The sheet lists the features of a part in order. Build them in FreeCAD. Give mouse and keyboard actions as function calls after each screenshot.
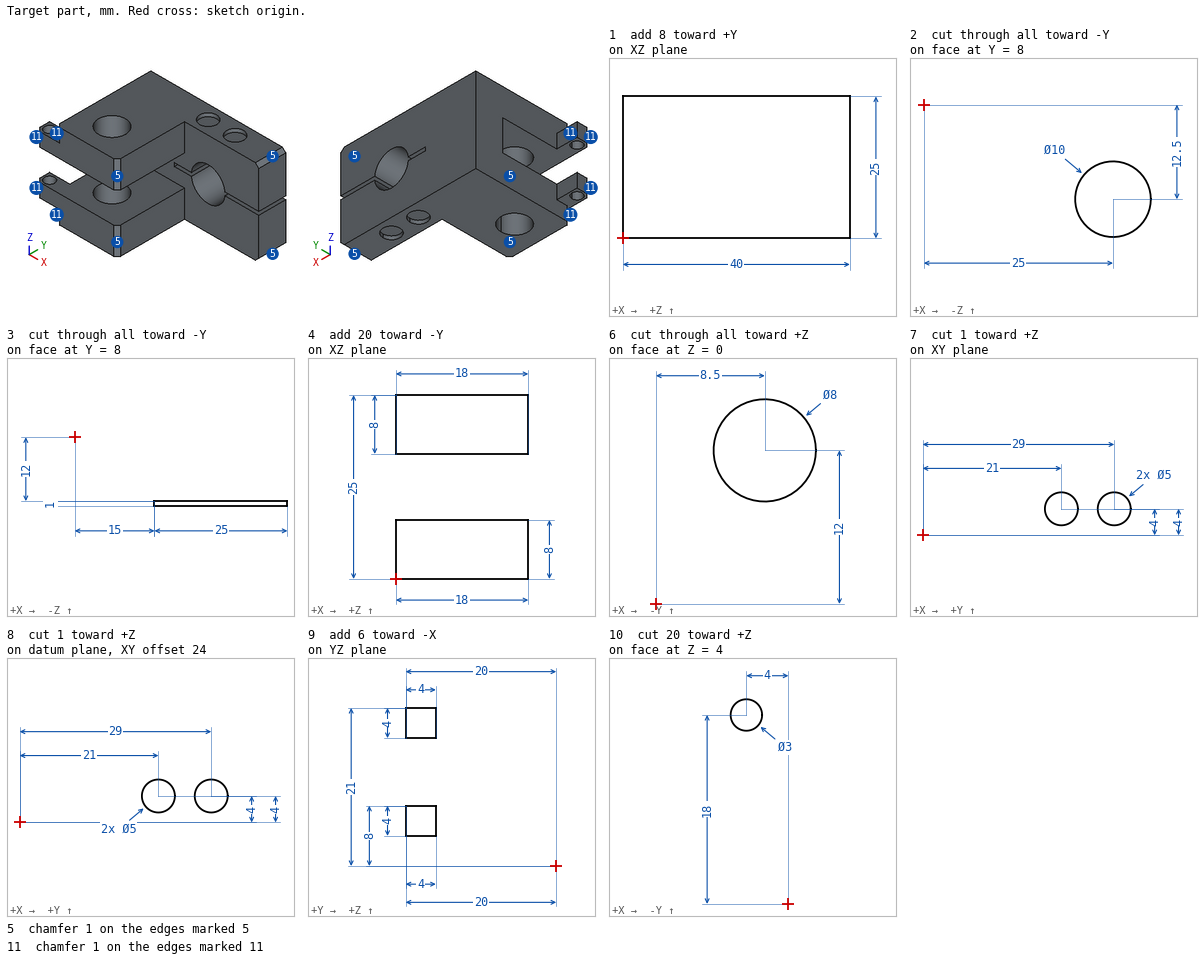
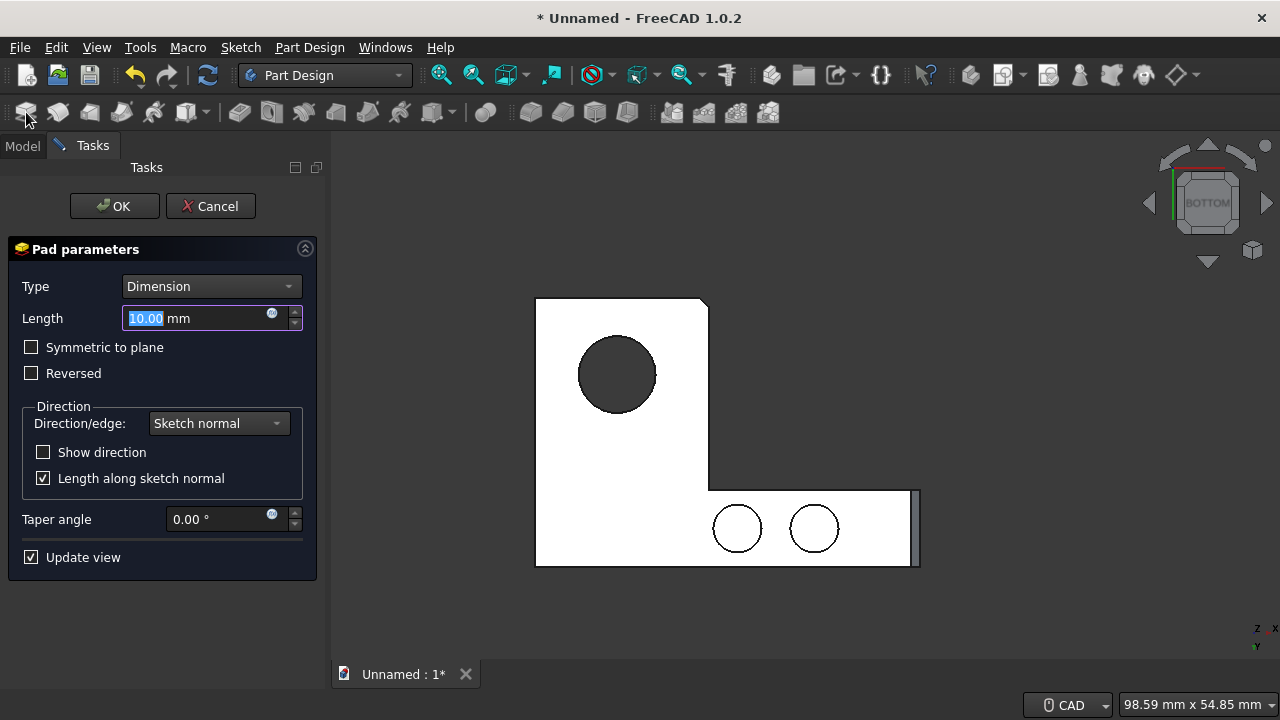
text(6)
key(Tab)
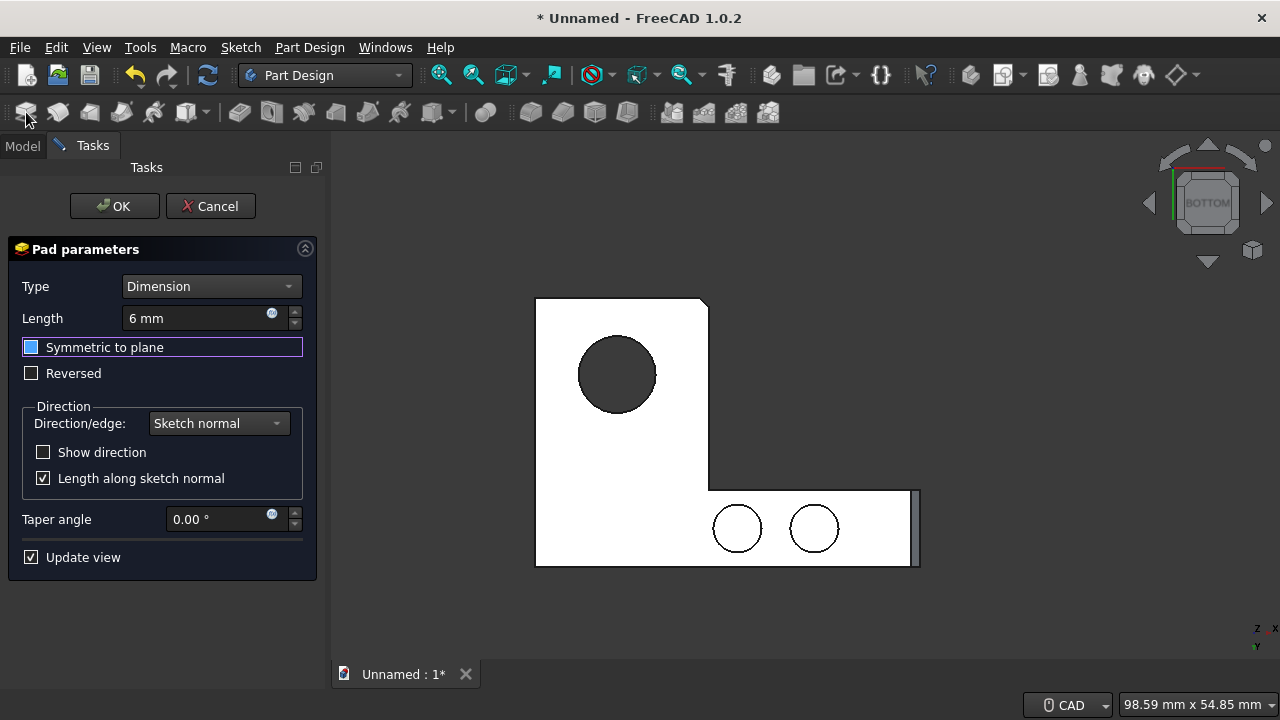
click(30, 373)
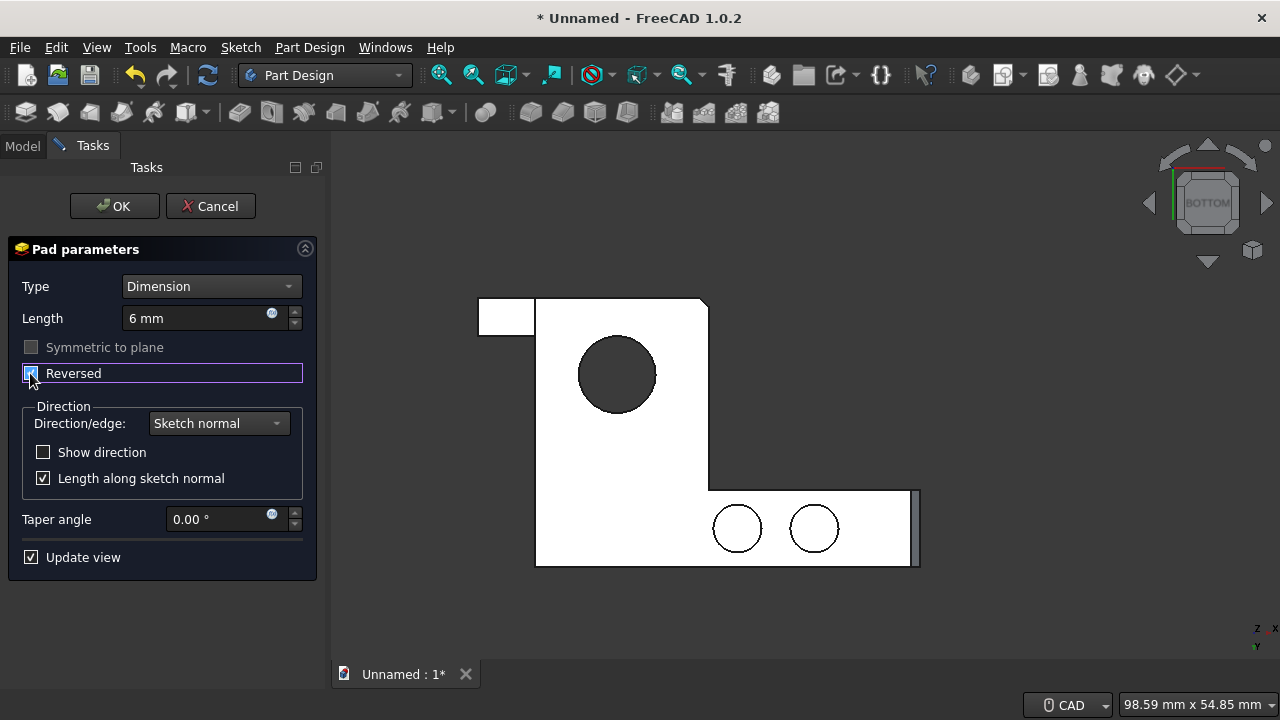
click(115, 206)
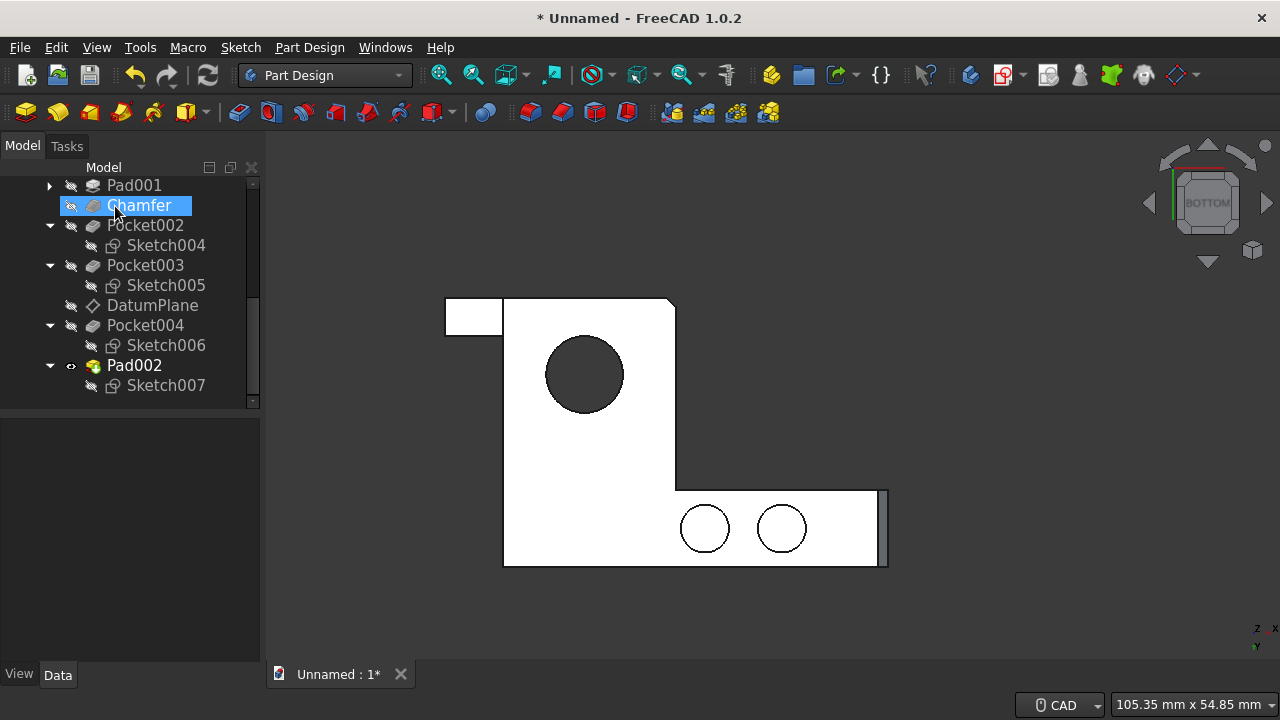
click(482, 316)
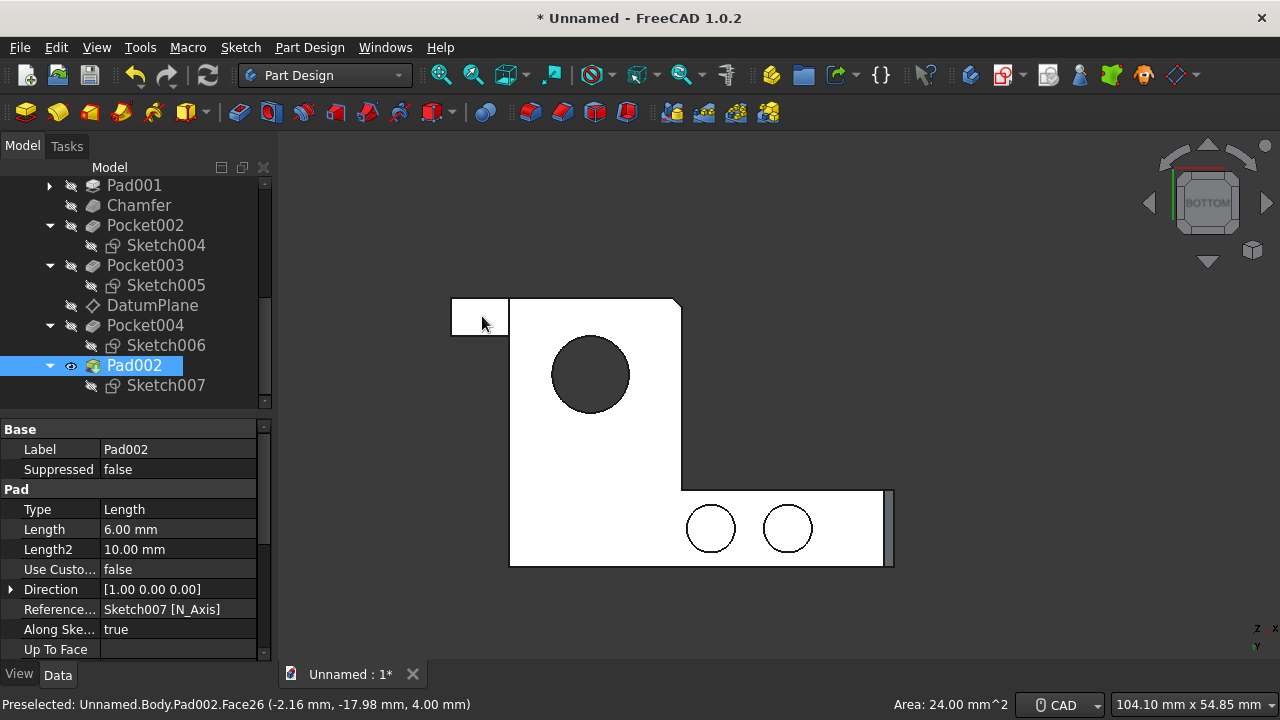
click(1004, 76)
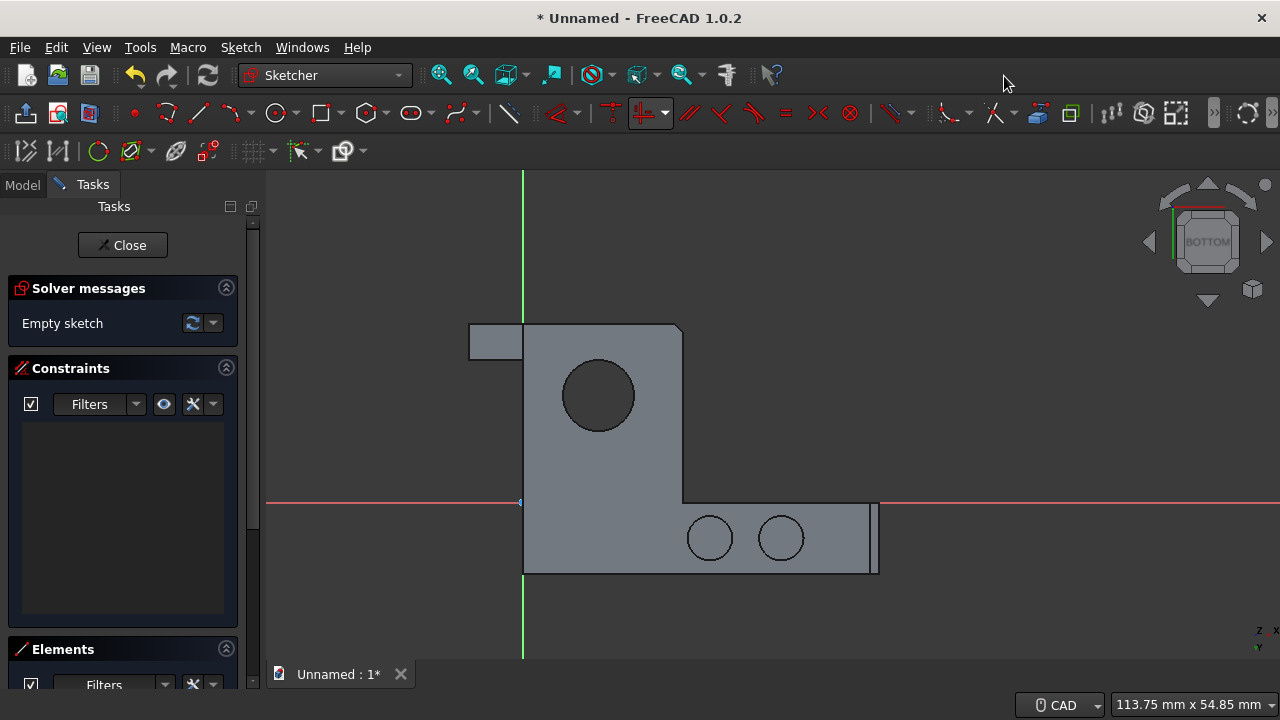
click(90, 114)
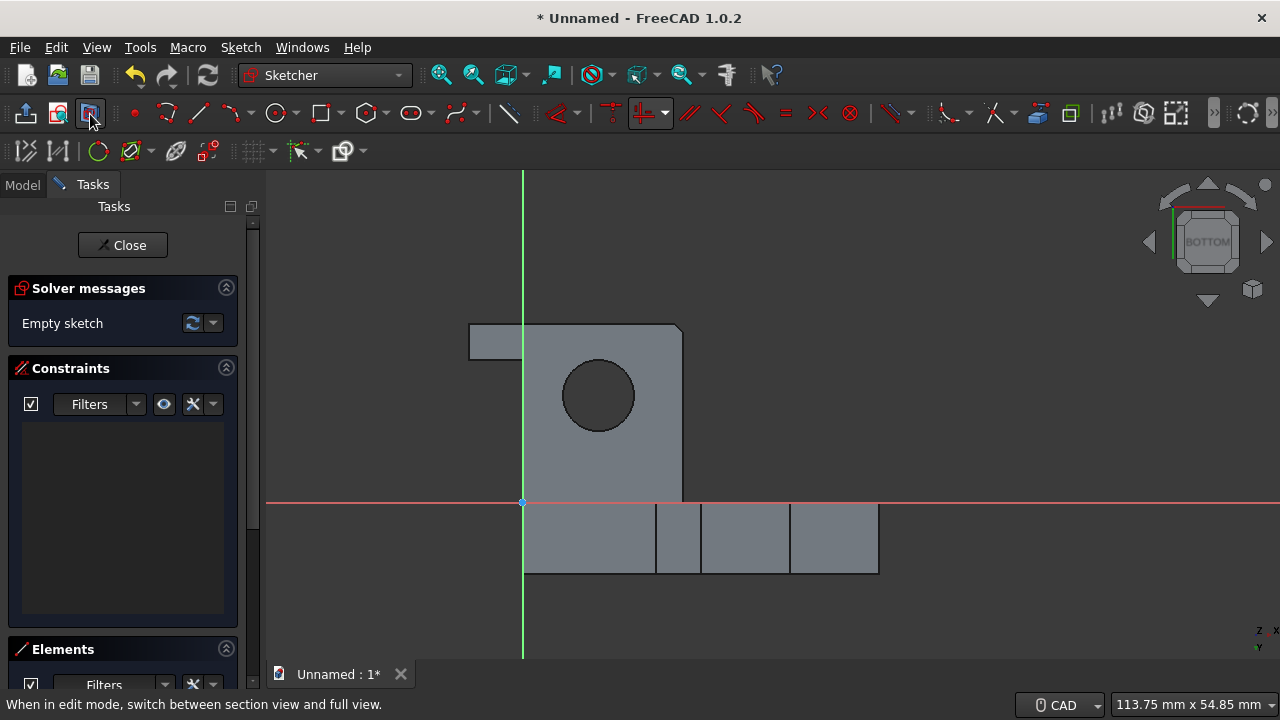
scroll(465, 335, up, 12)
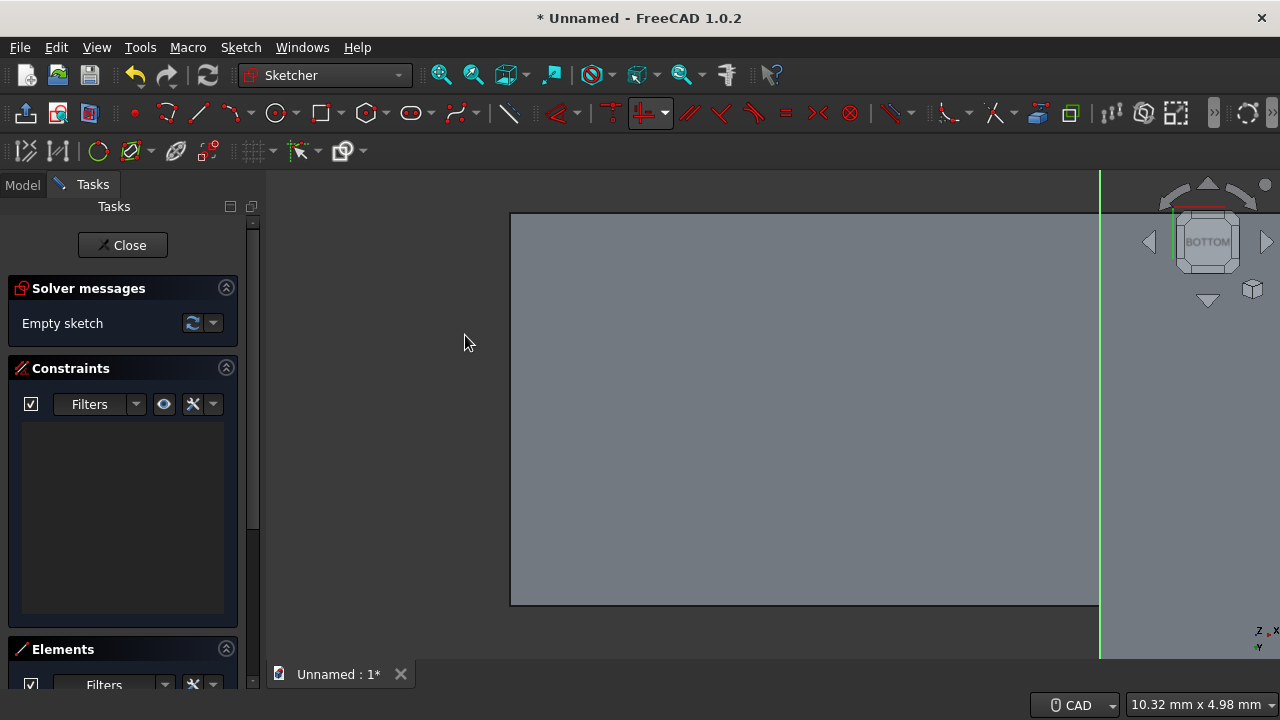
click(276, 114)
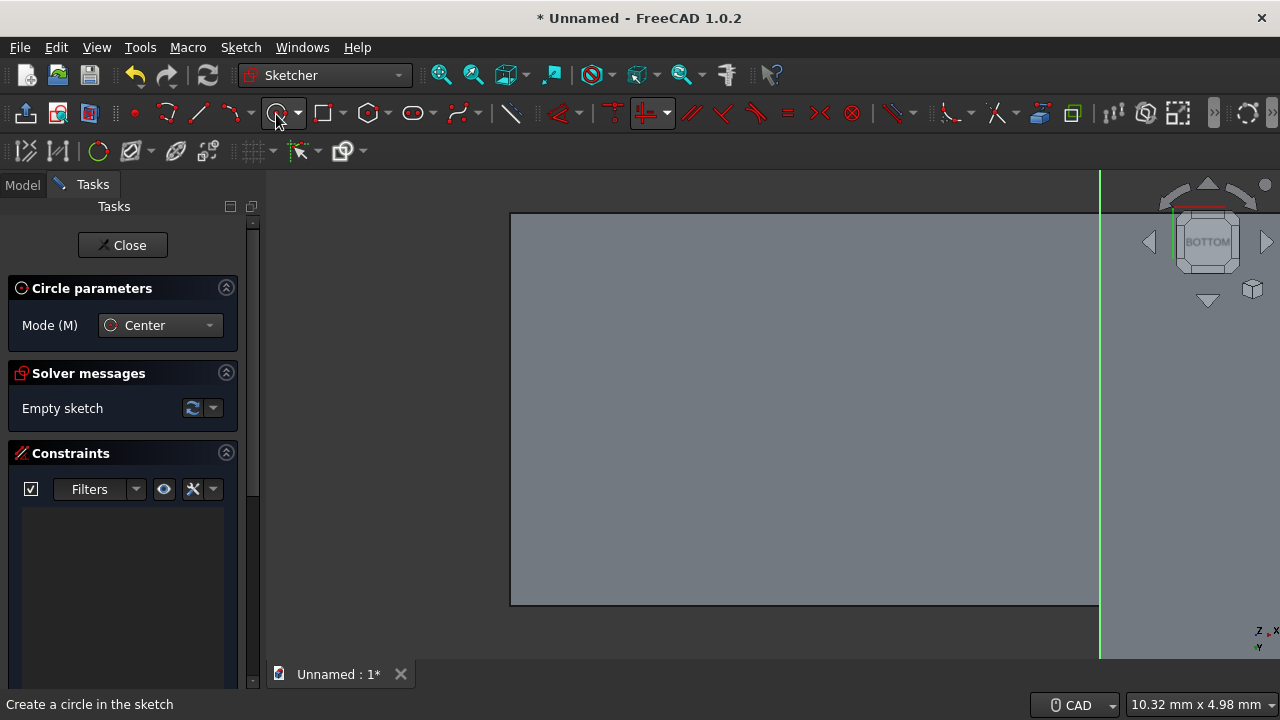
click(707, 409)
click(811, 305)
key(Escape)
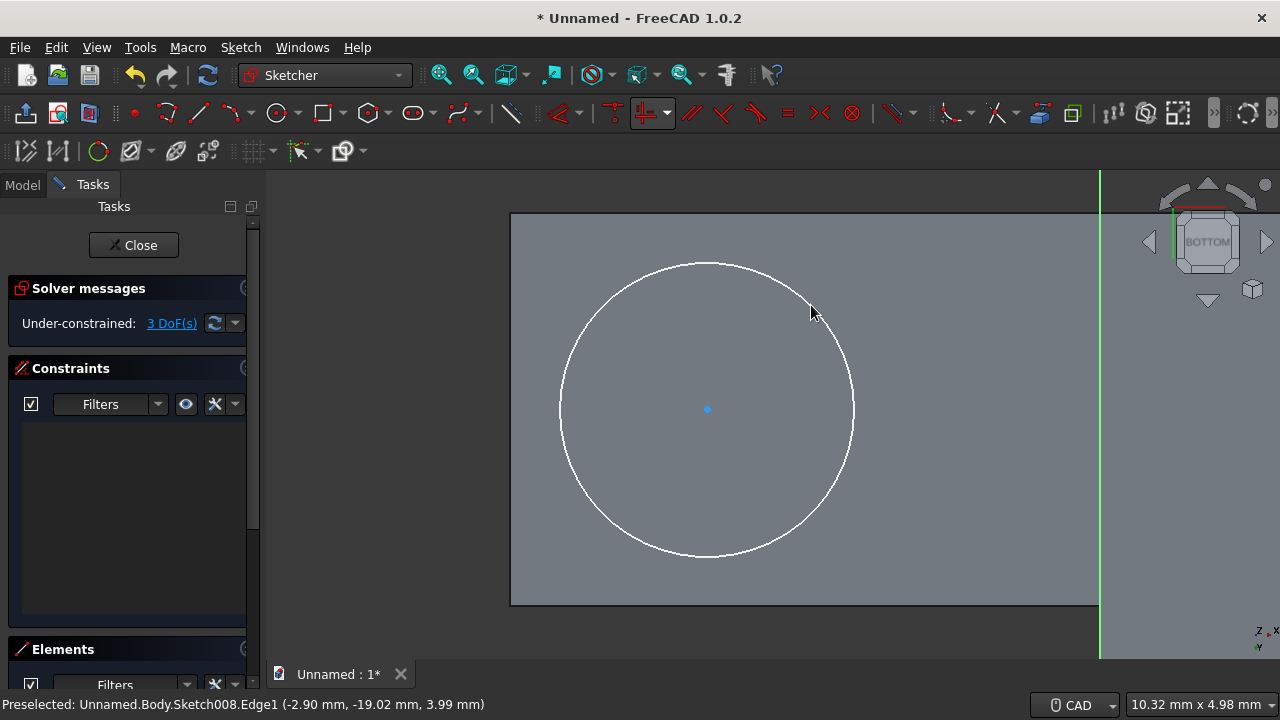
click(558, 114)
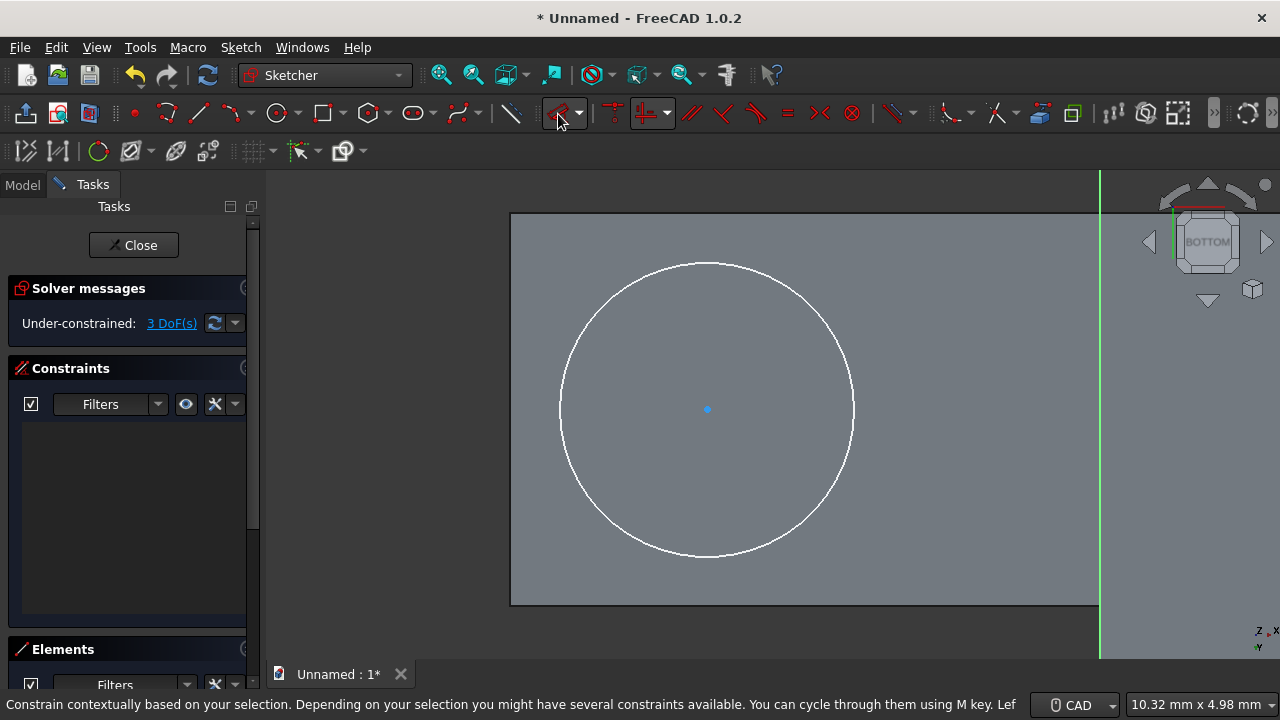
click(811, 306)
click(834, 283)